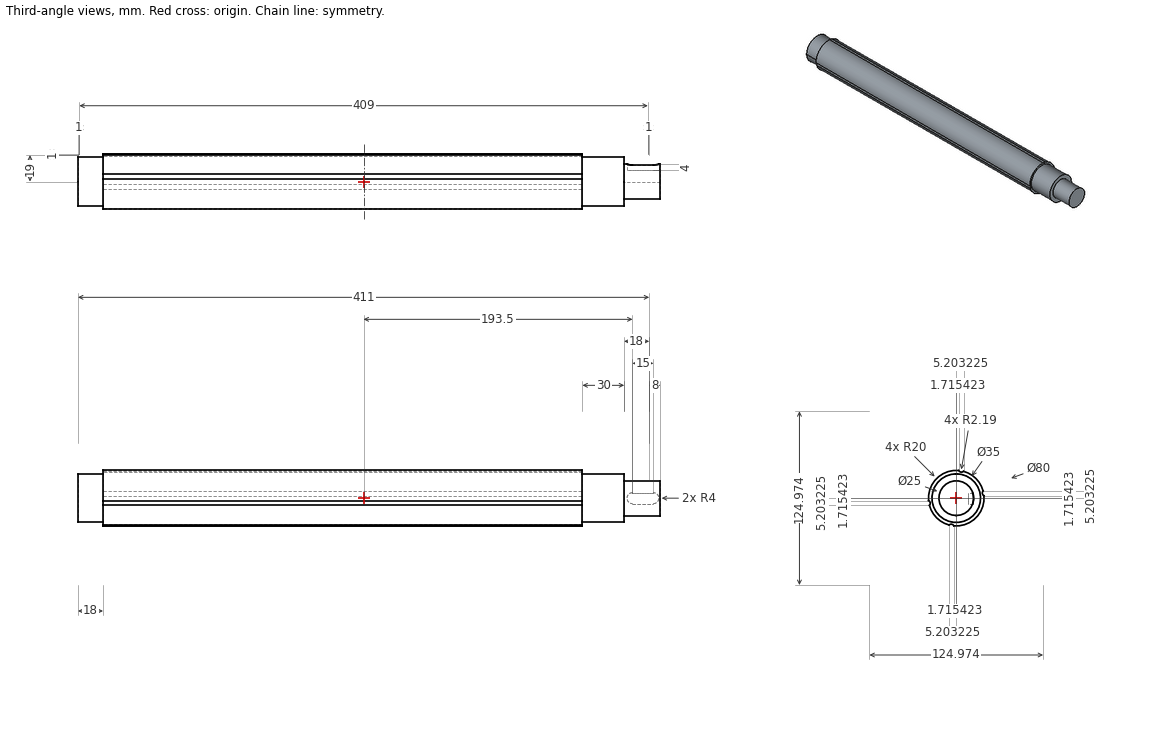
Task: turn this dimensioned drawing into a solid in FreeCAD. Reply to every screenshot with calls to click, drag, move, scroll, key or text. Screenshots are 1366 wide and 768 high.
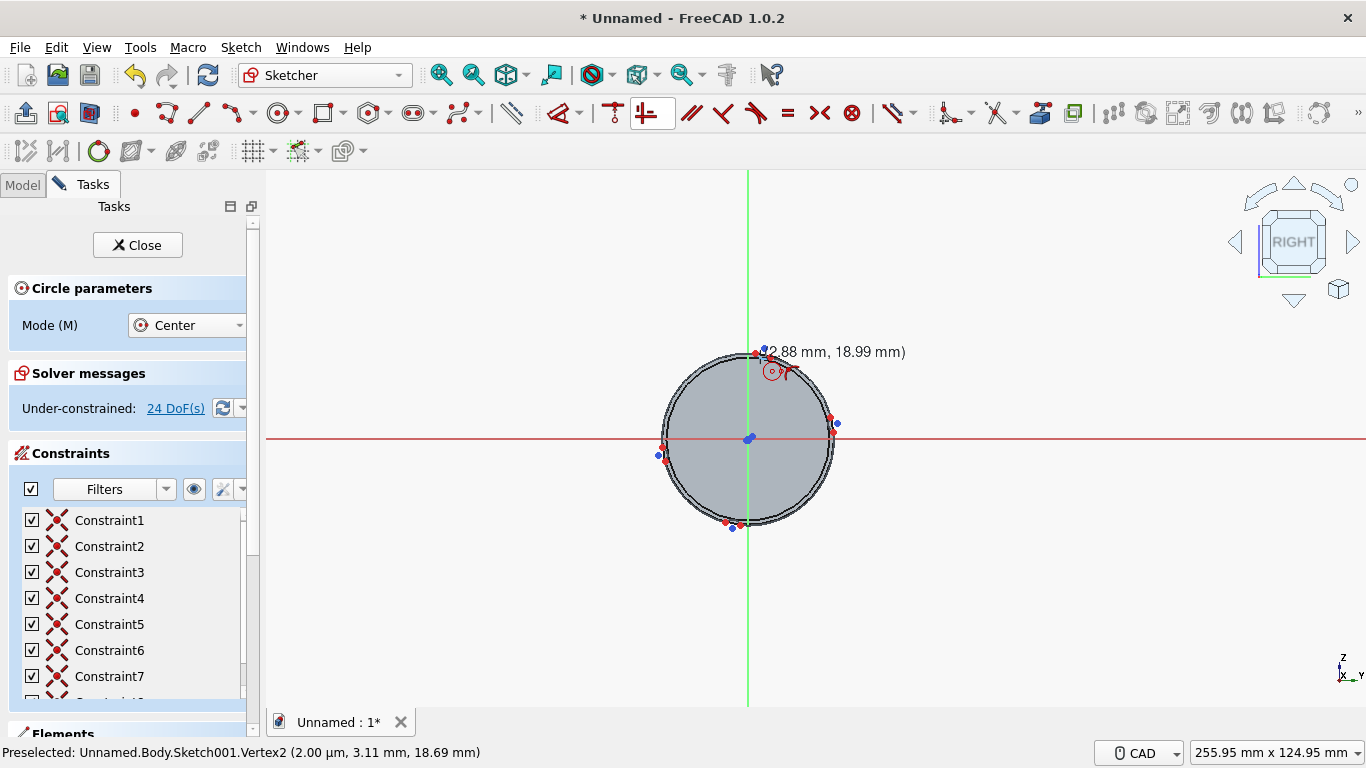
click(748, 439)
click(870, 318)
key(Escape)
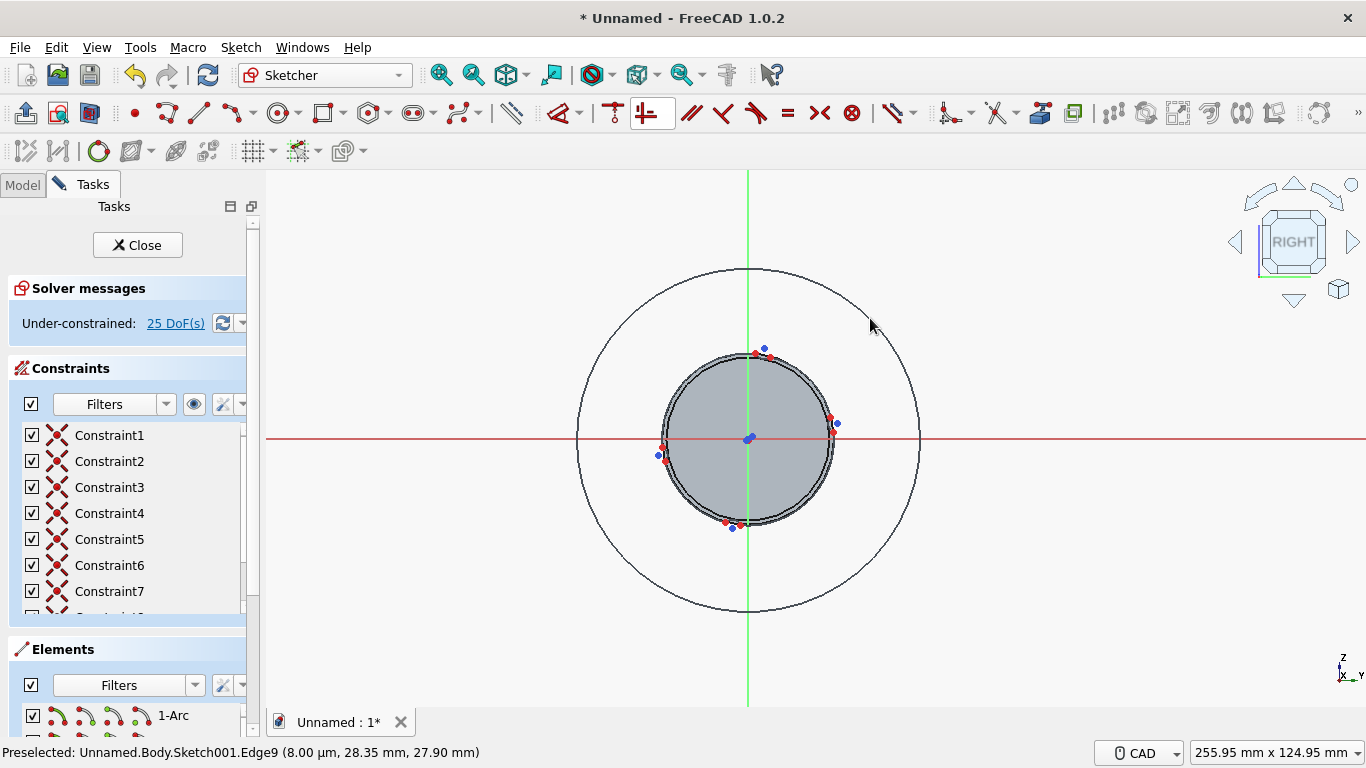
click(870, 319)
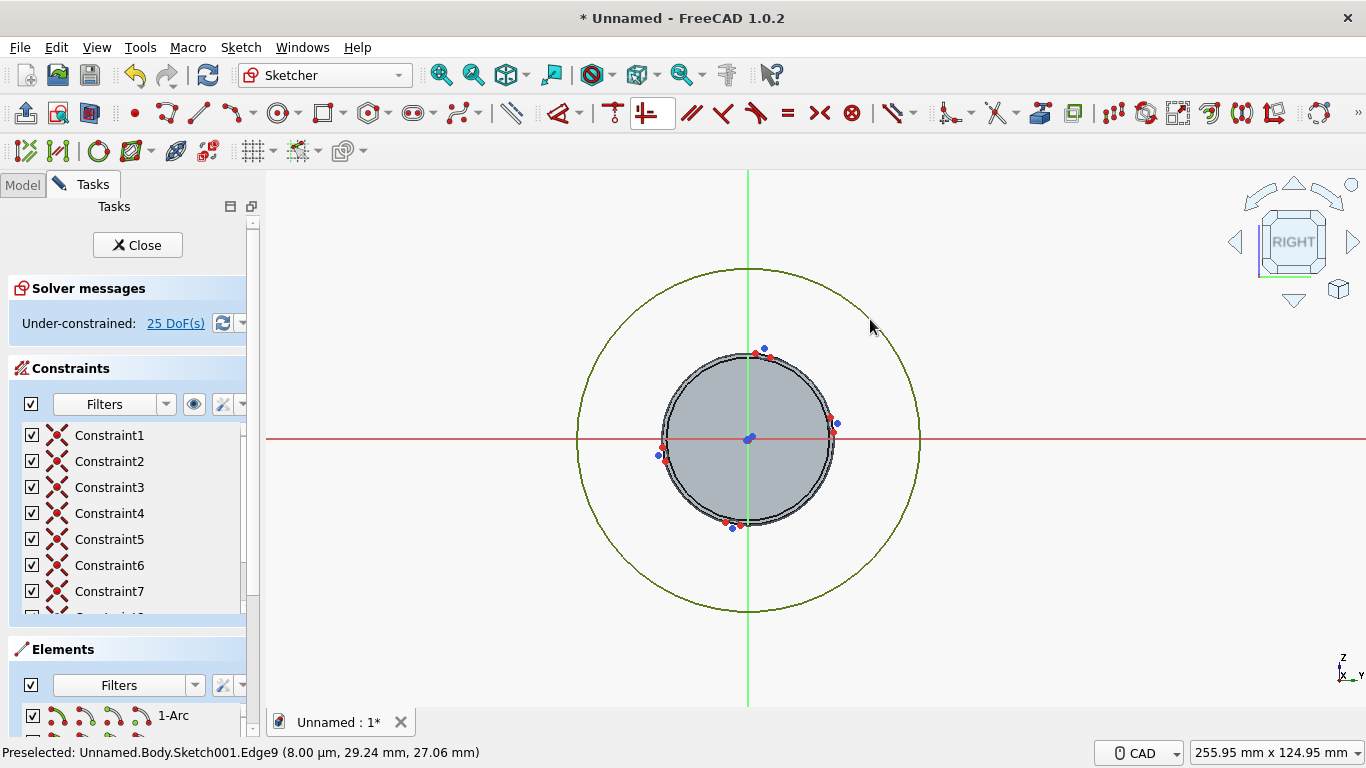
click(820, 393)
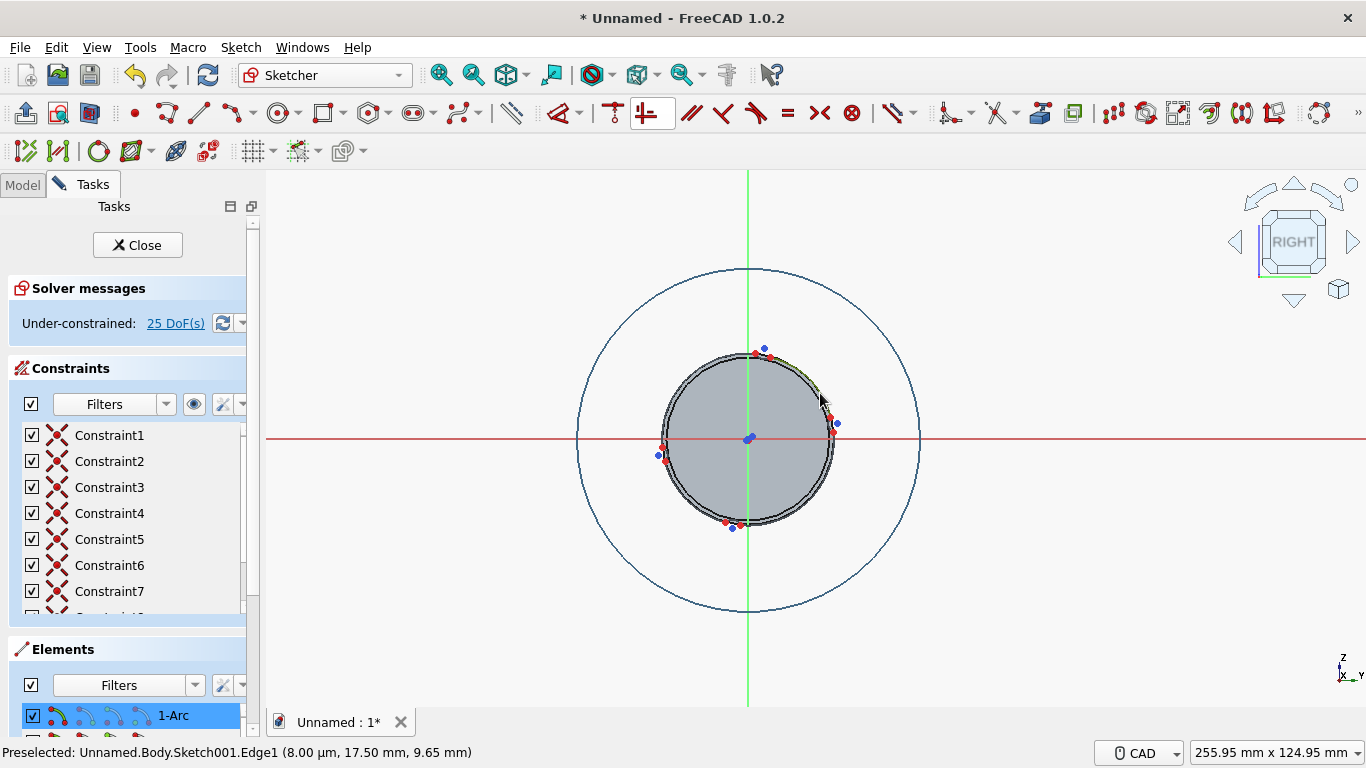
key(c)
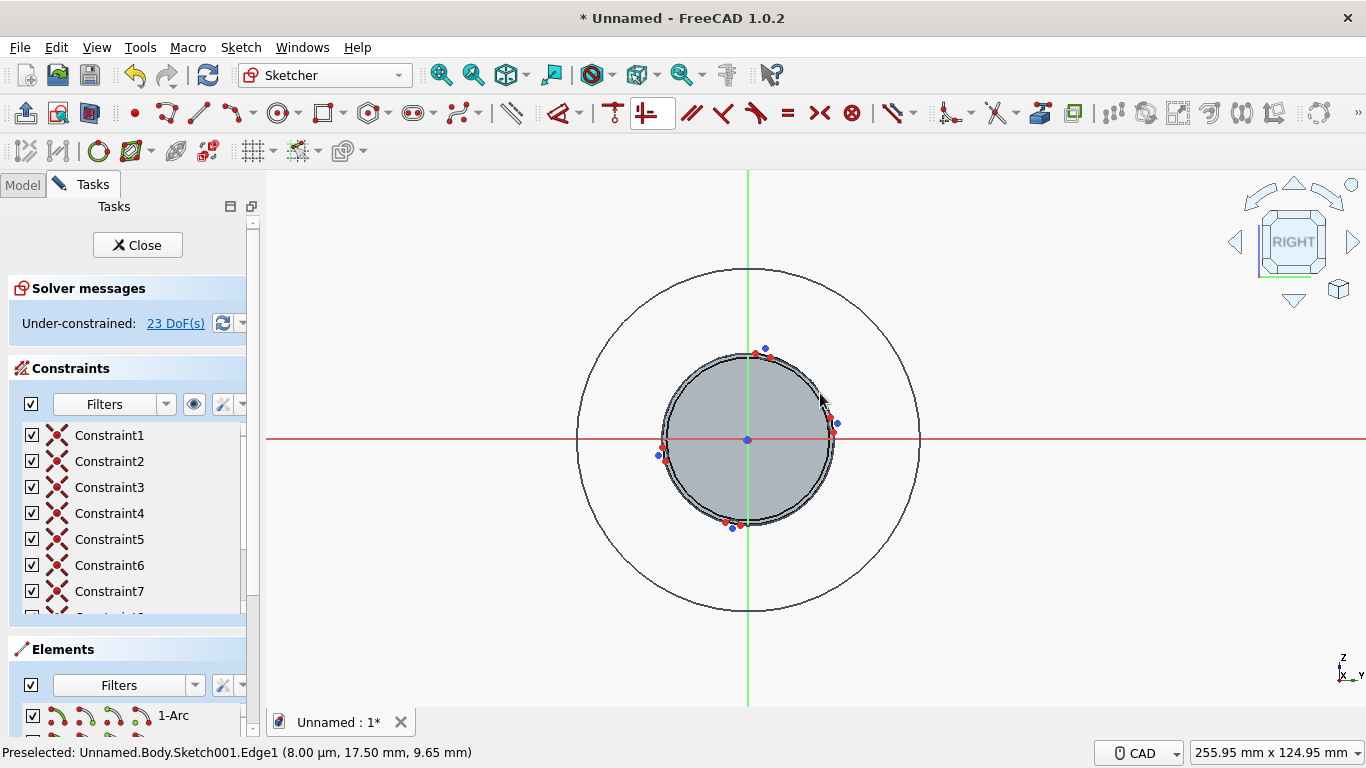
click(869, 318)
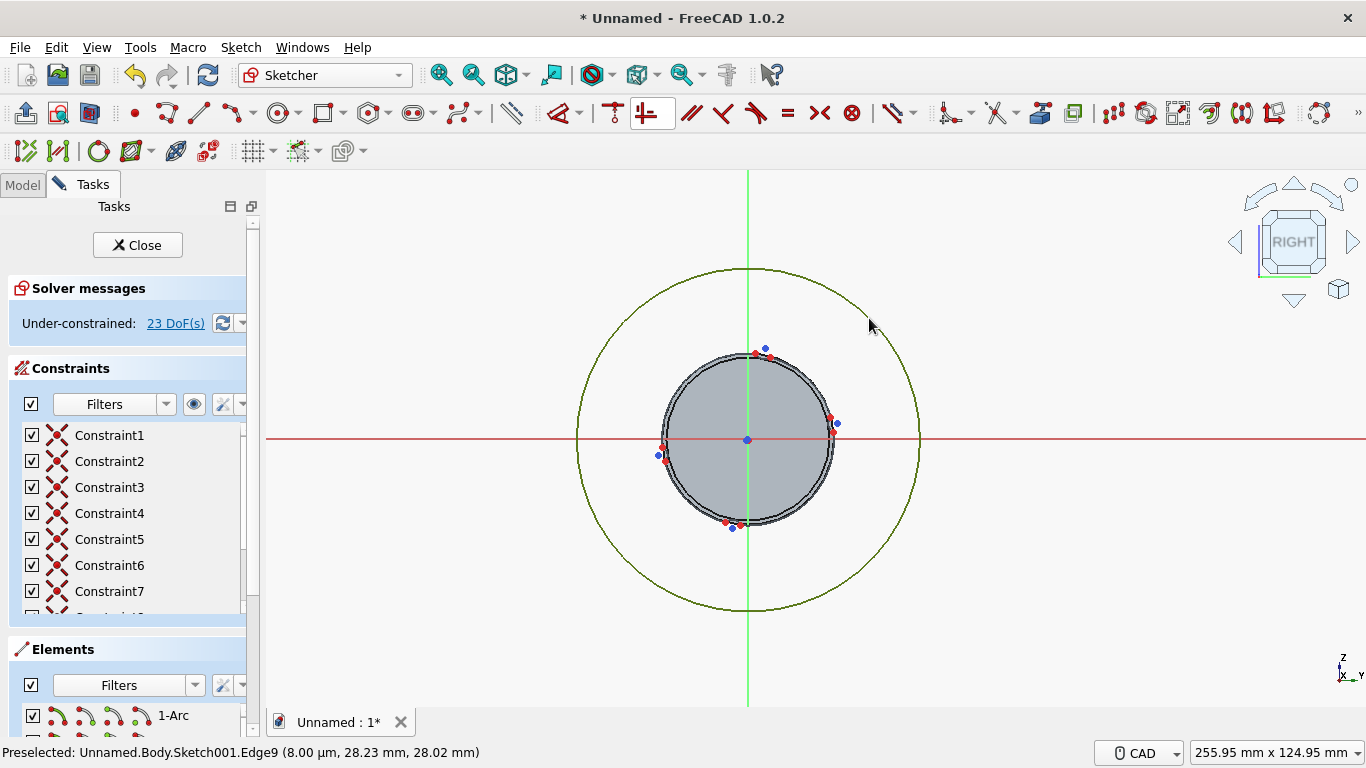
click(676, 487)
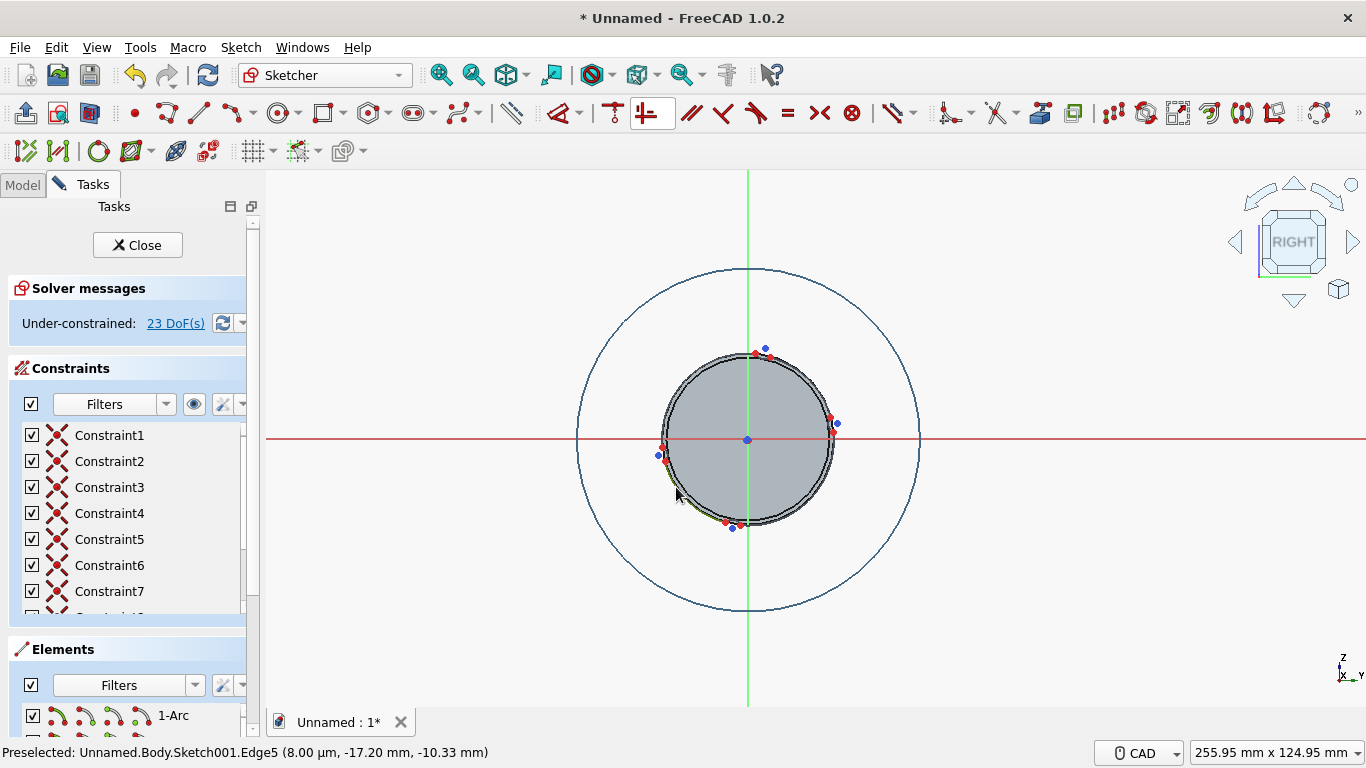
key(c)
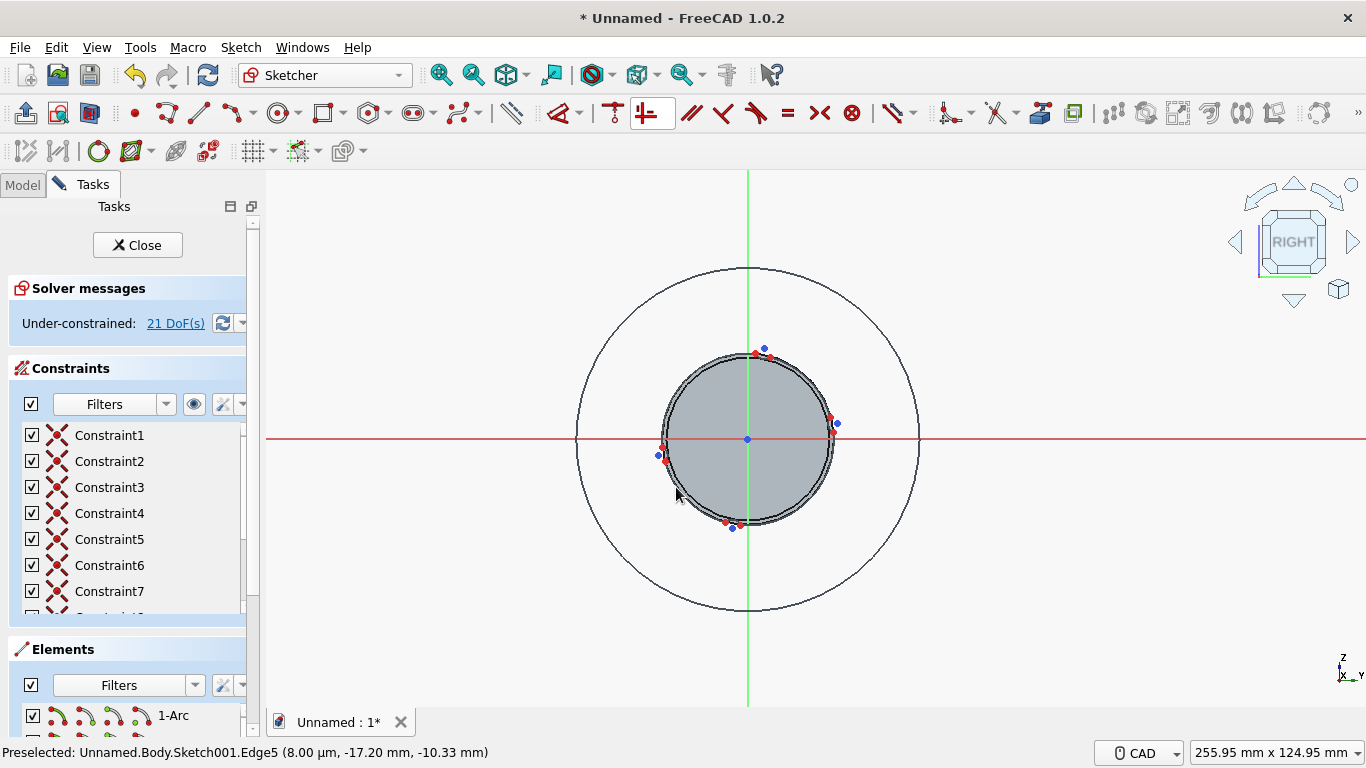
click(869, 318)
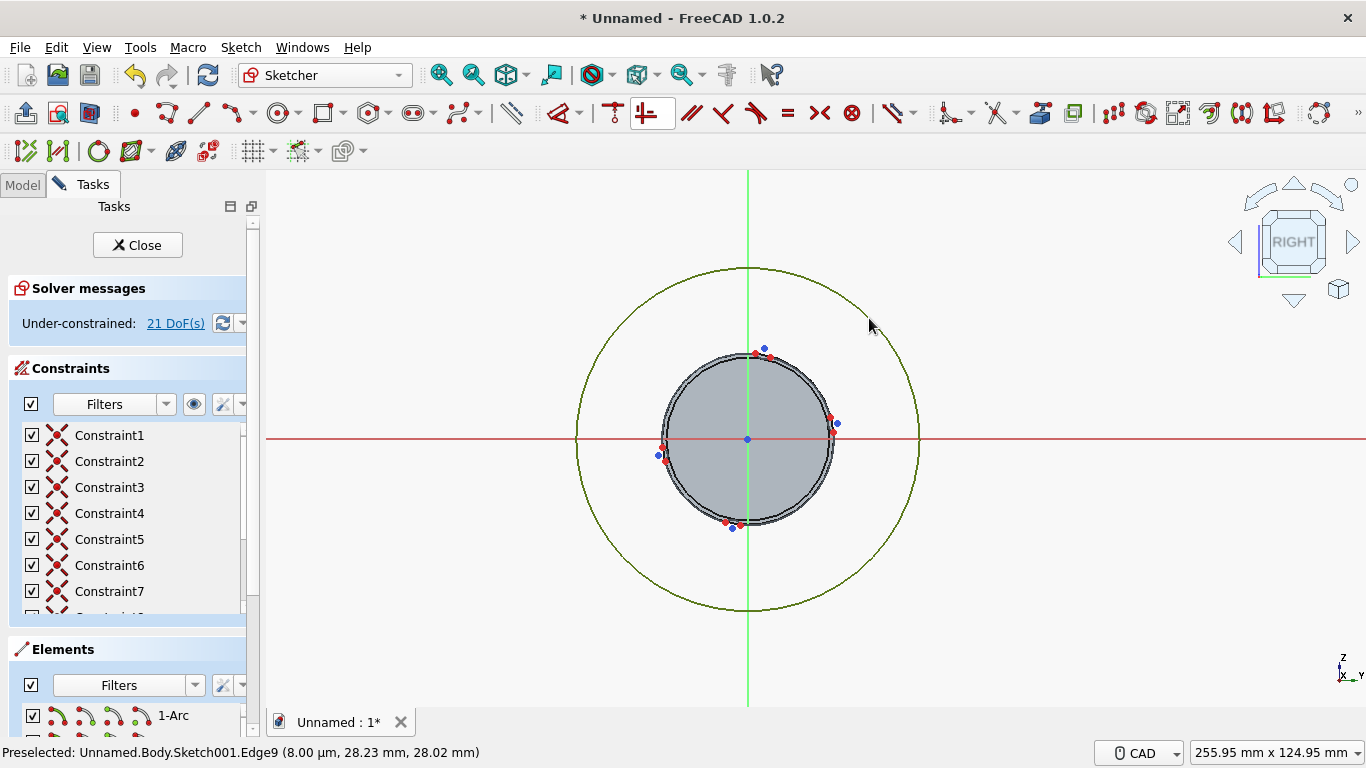
click(712, 362)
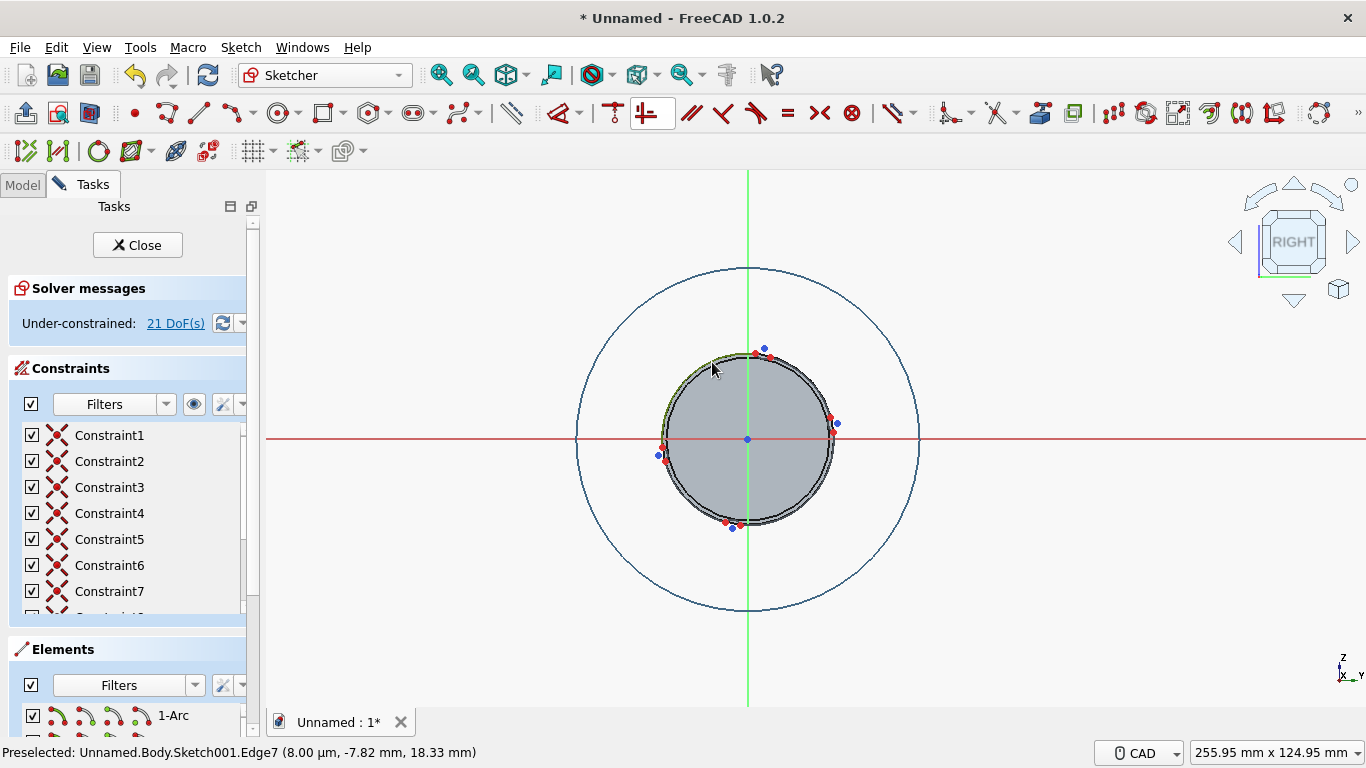
click(614, 114)